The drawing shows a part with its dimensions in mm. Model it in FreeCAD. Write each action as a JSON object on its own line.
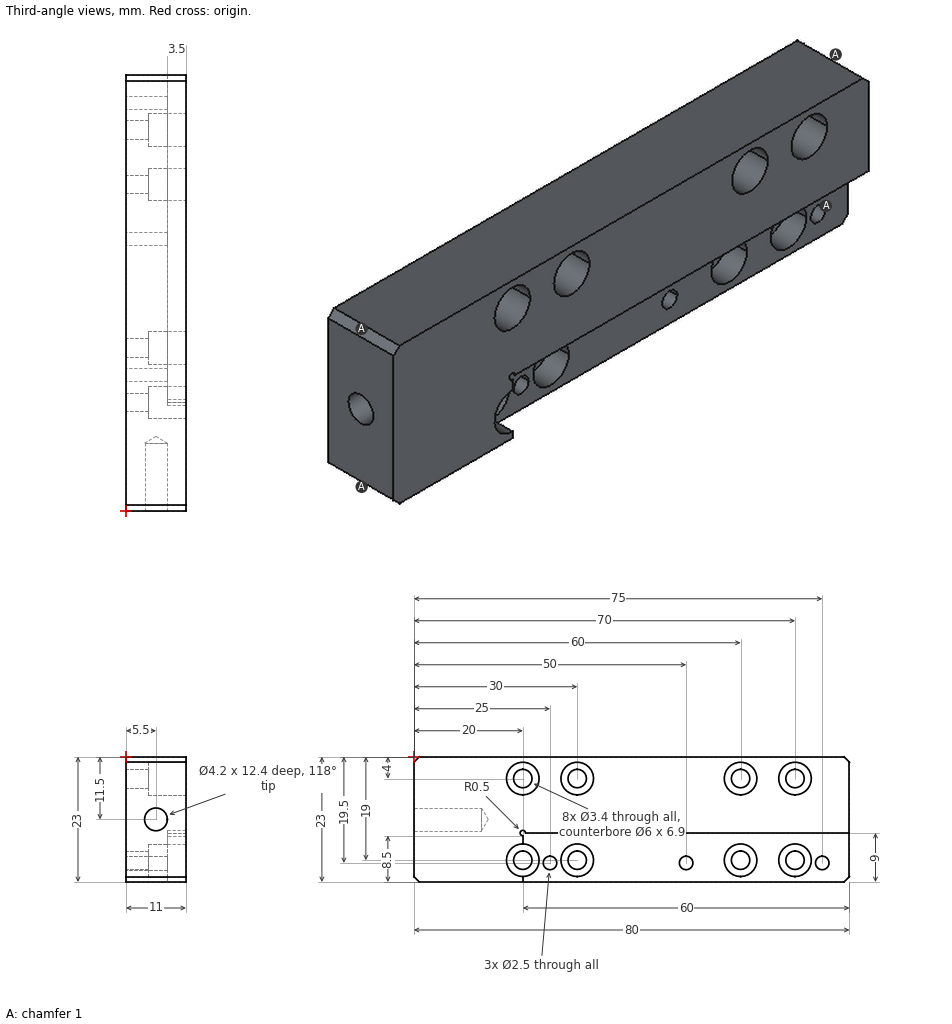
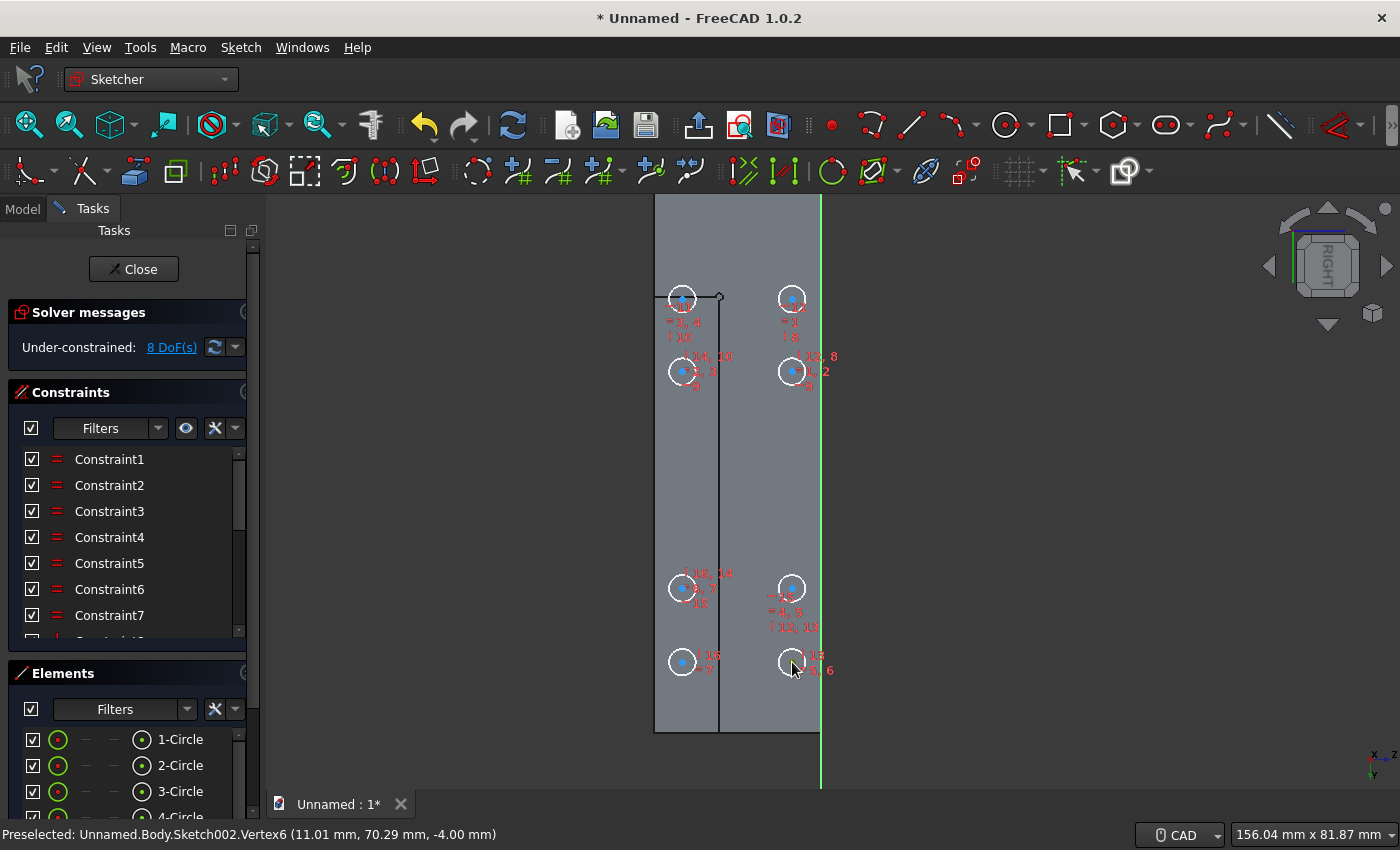
{"action": "left_click", "coordinate": [682, 662]}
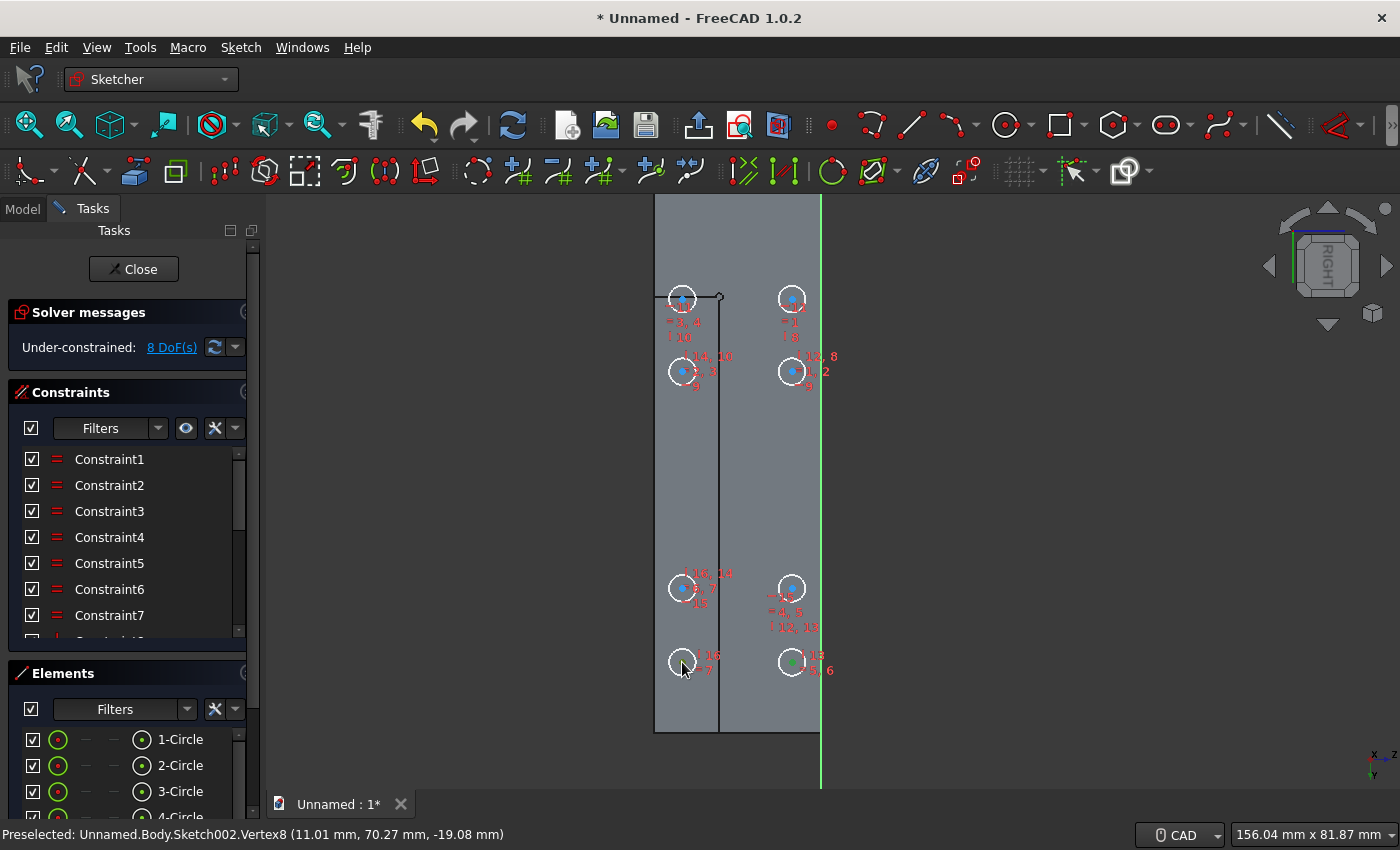
{"action": "key", "text": "h"}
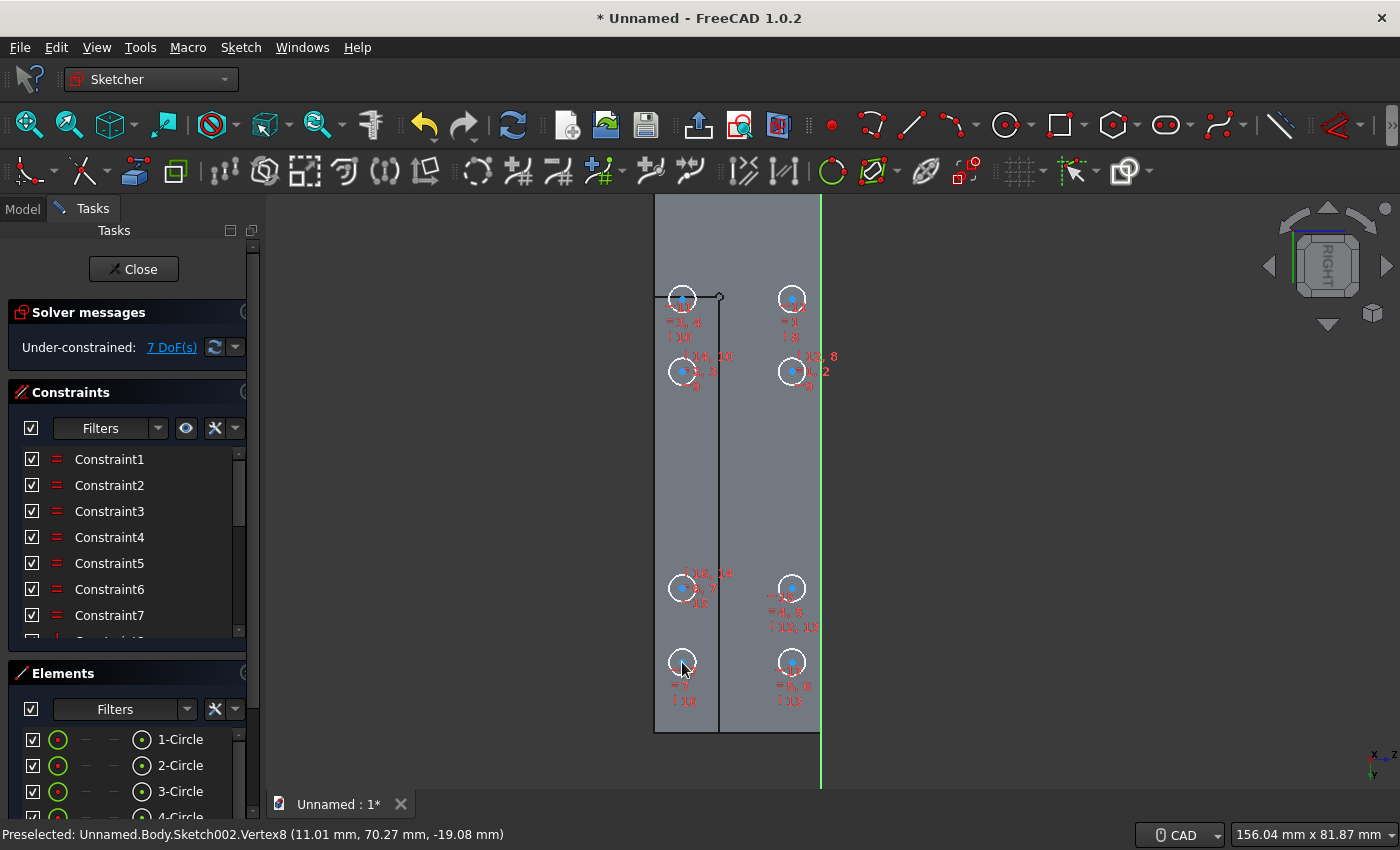
{"action": "left_click", "coordinate": [1336, 126]}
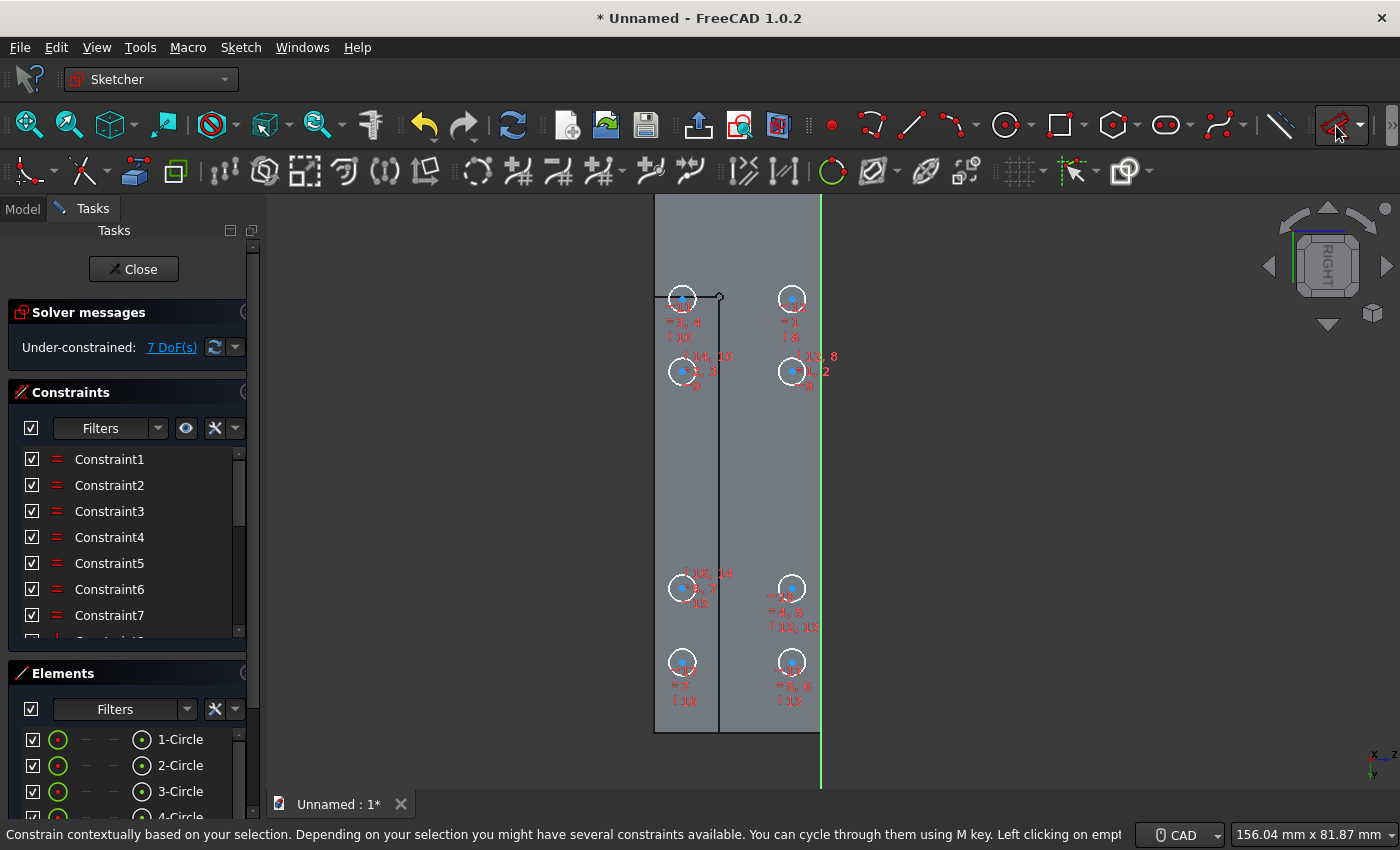
{"action": "scroll", "coordinate": [801, 290], "scroll_direction": "up", "scroll_amount": 3}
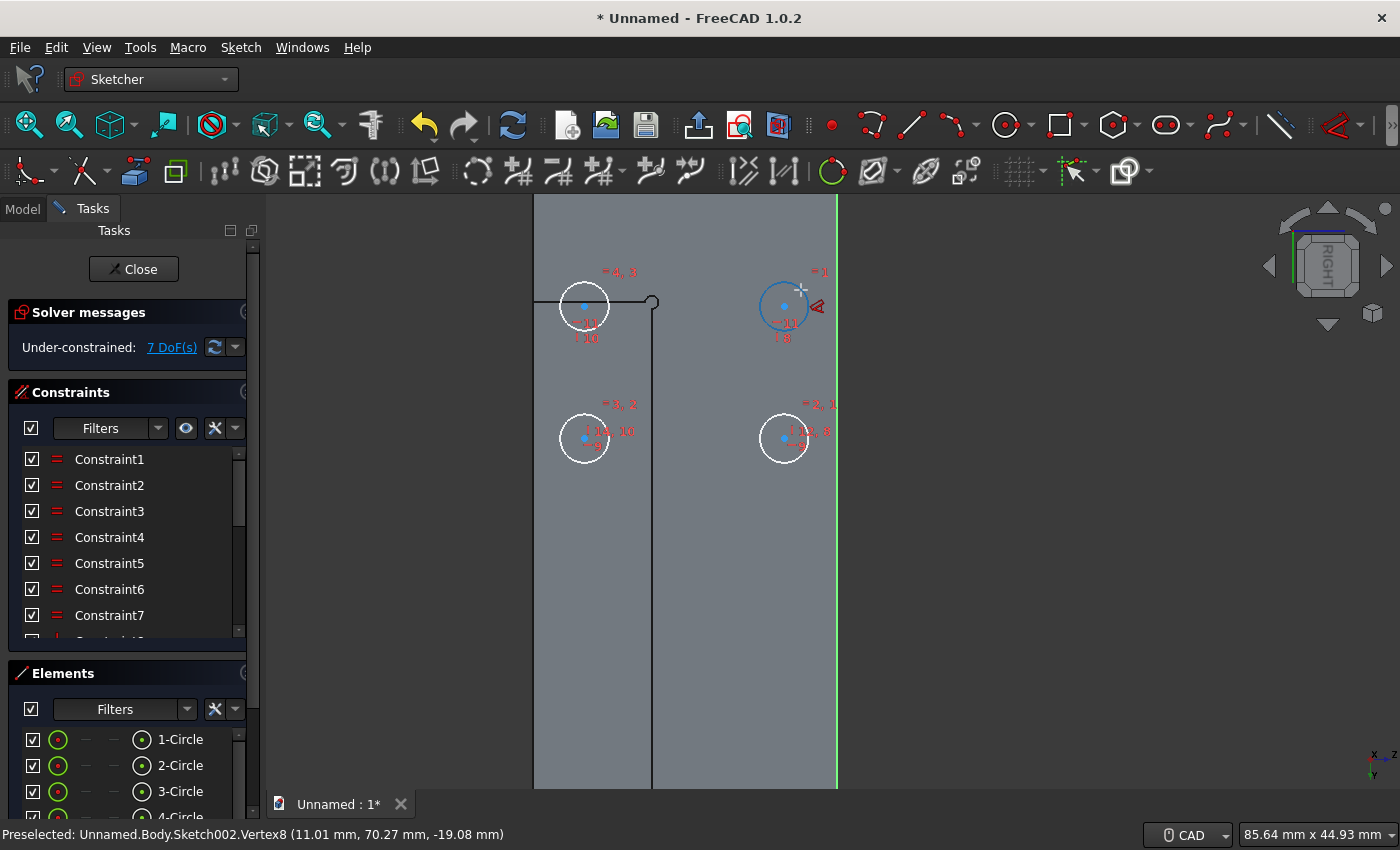
{"action": "left_click", "coordinate": [801, 289]}
{"action": "left_click", "coordinate": [823, 266]}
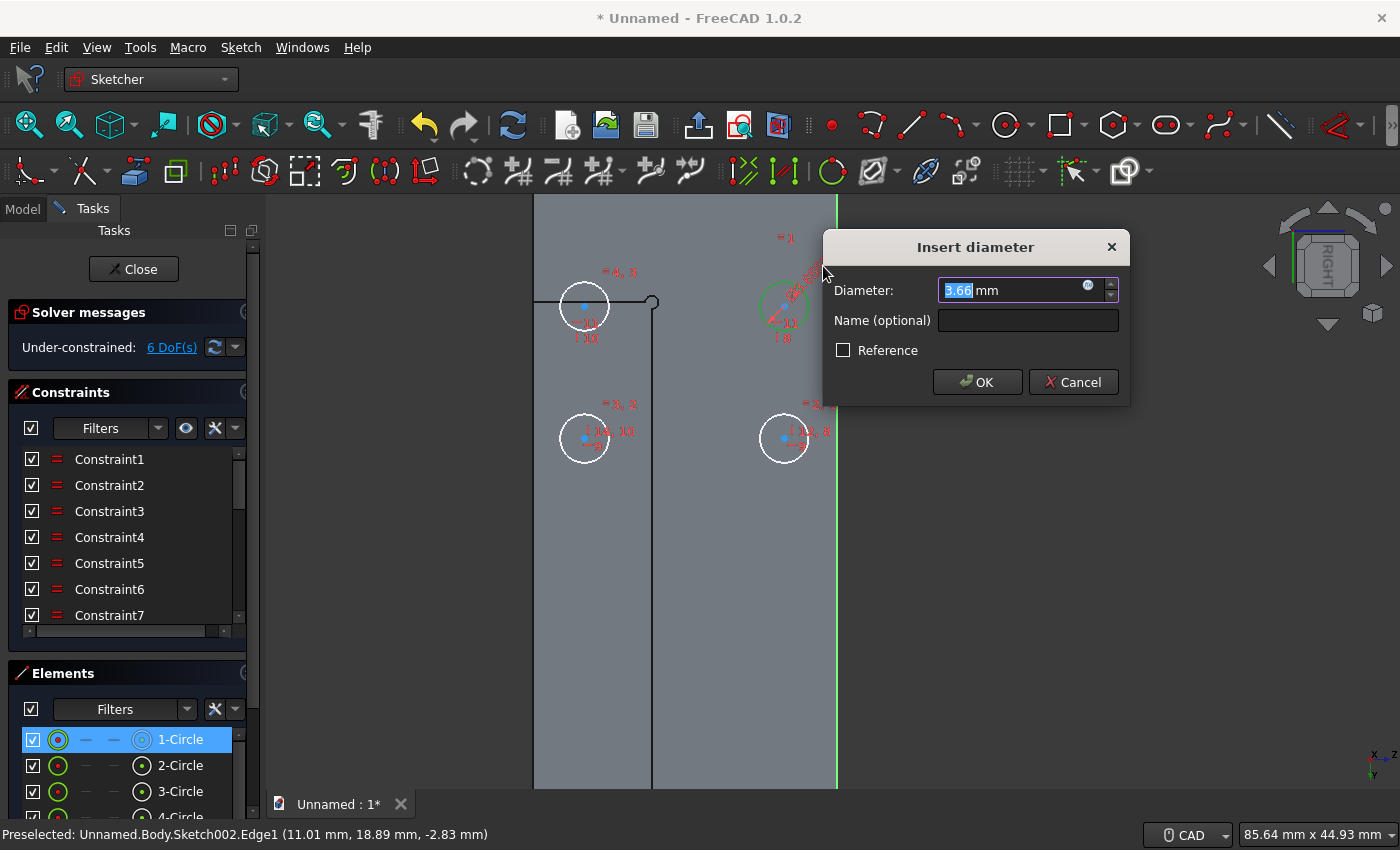
{"action": "type", "text": "3.4"}
{"action": "key", "text": "Return"}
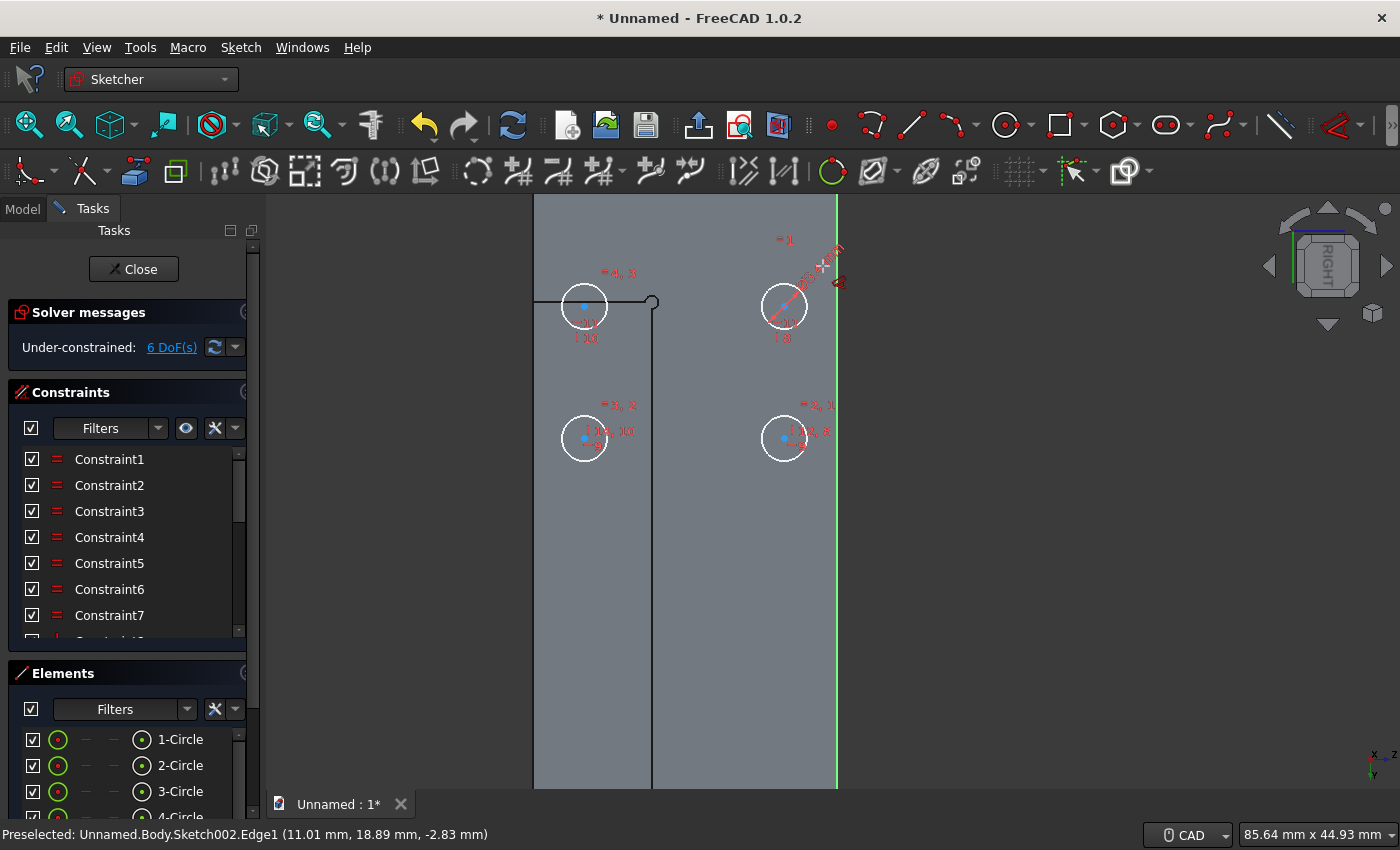
{"action": "left_click", "coordinate": [784, 306]}
{"action": "left_click", "coordinate": [811, 340]}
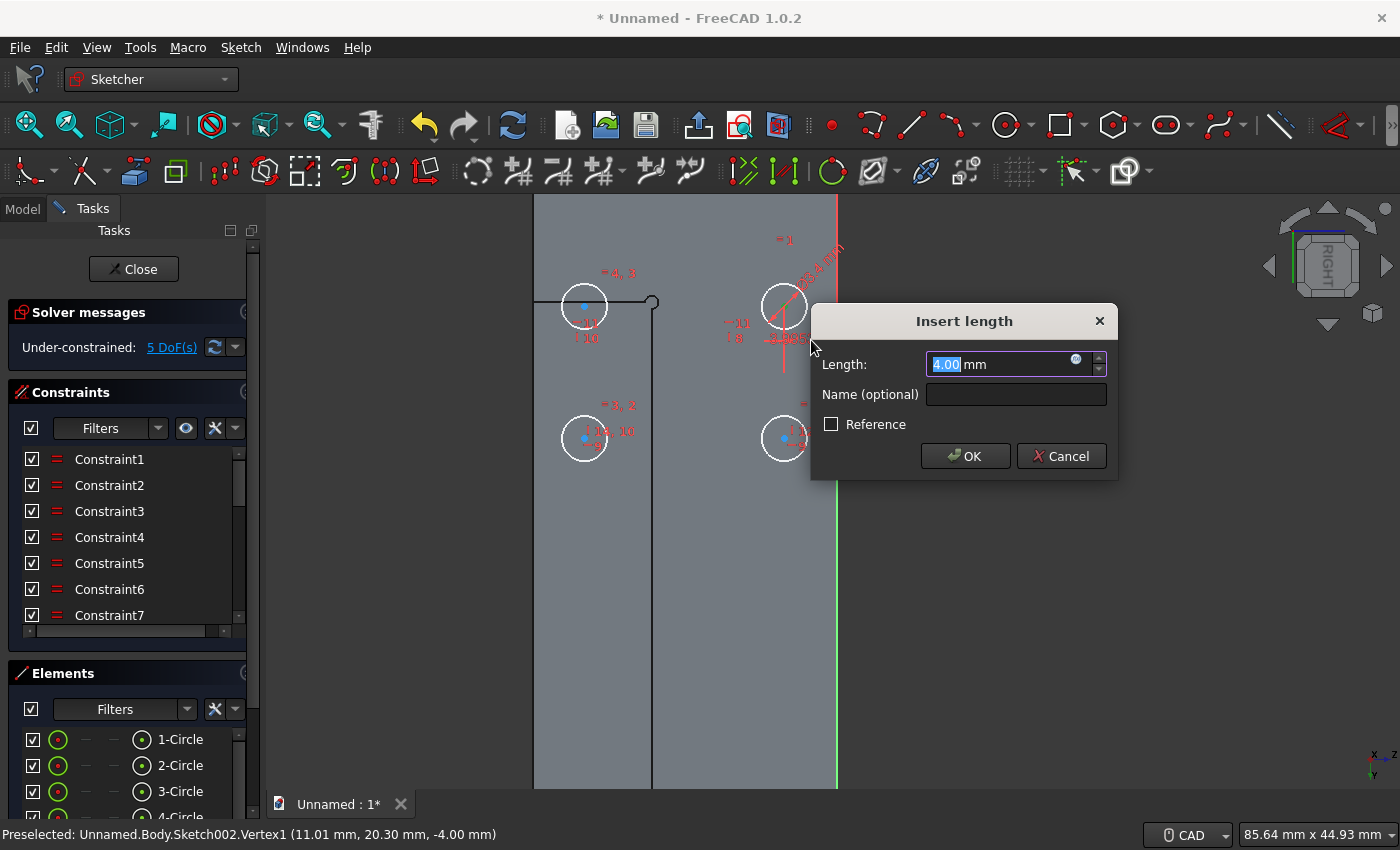
{"action": "type", "text": "4"}
{"action": "key", "text": "Return"}